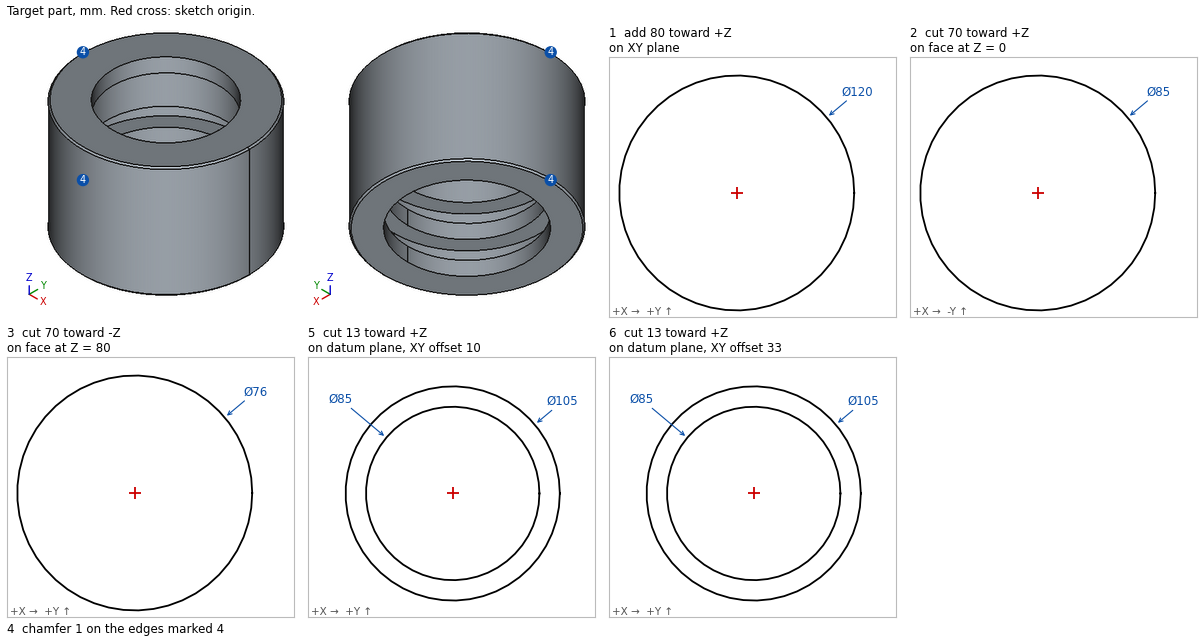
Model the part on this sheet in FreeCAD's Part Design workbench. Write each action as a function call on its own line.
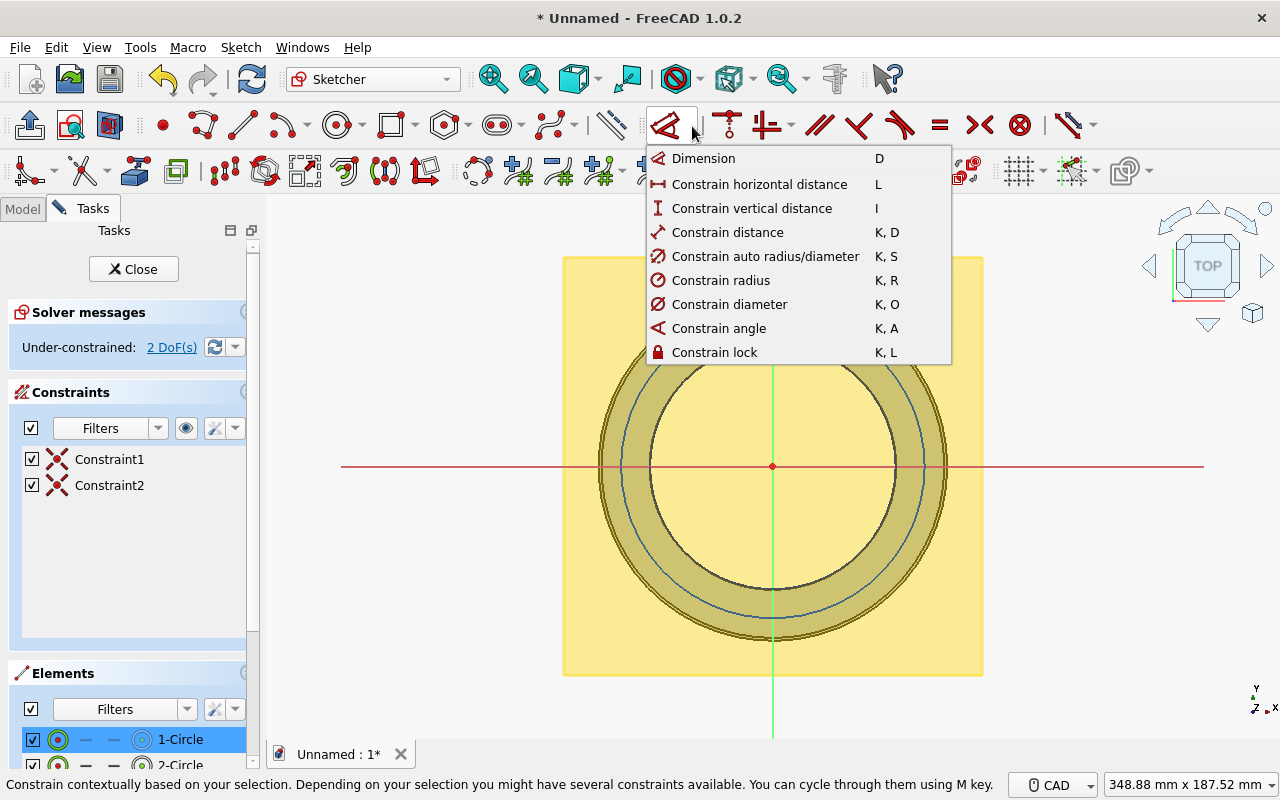
click(799, 304)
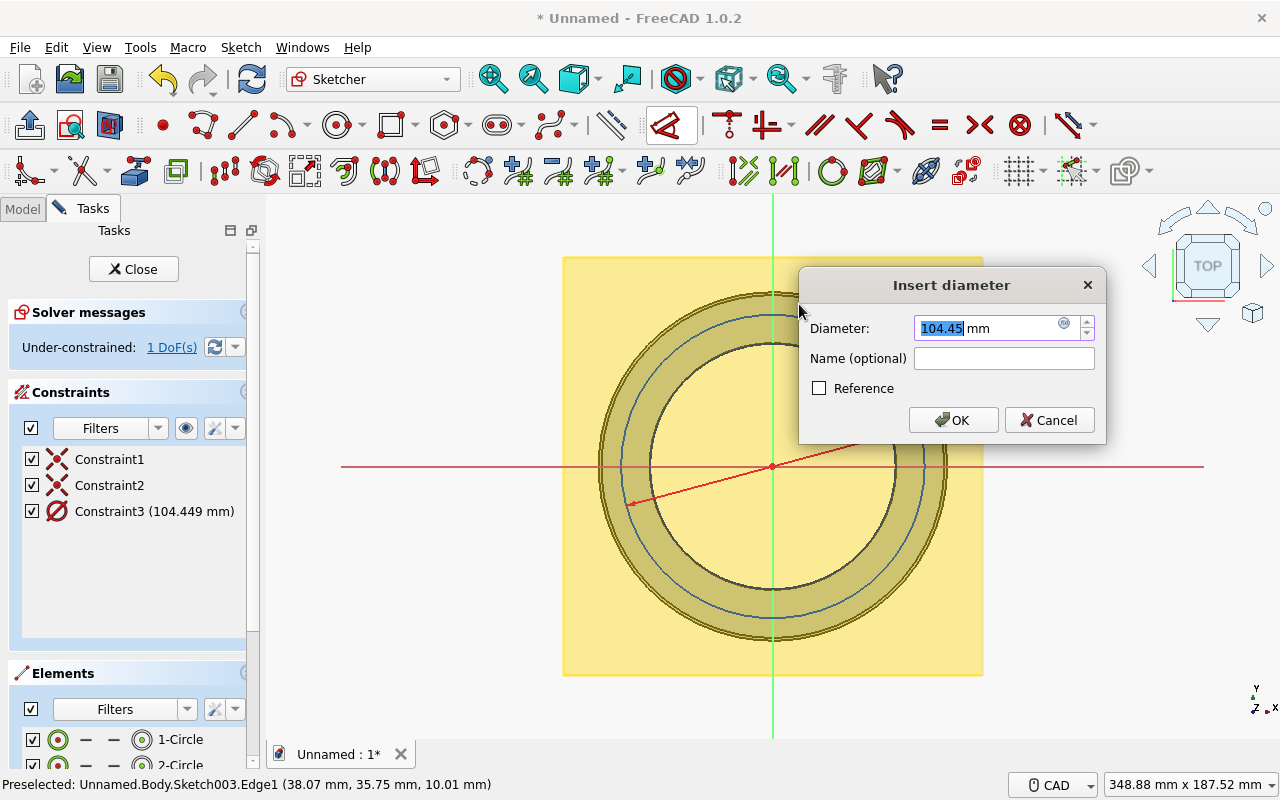
text(105)
key(Return)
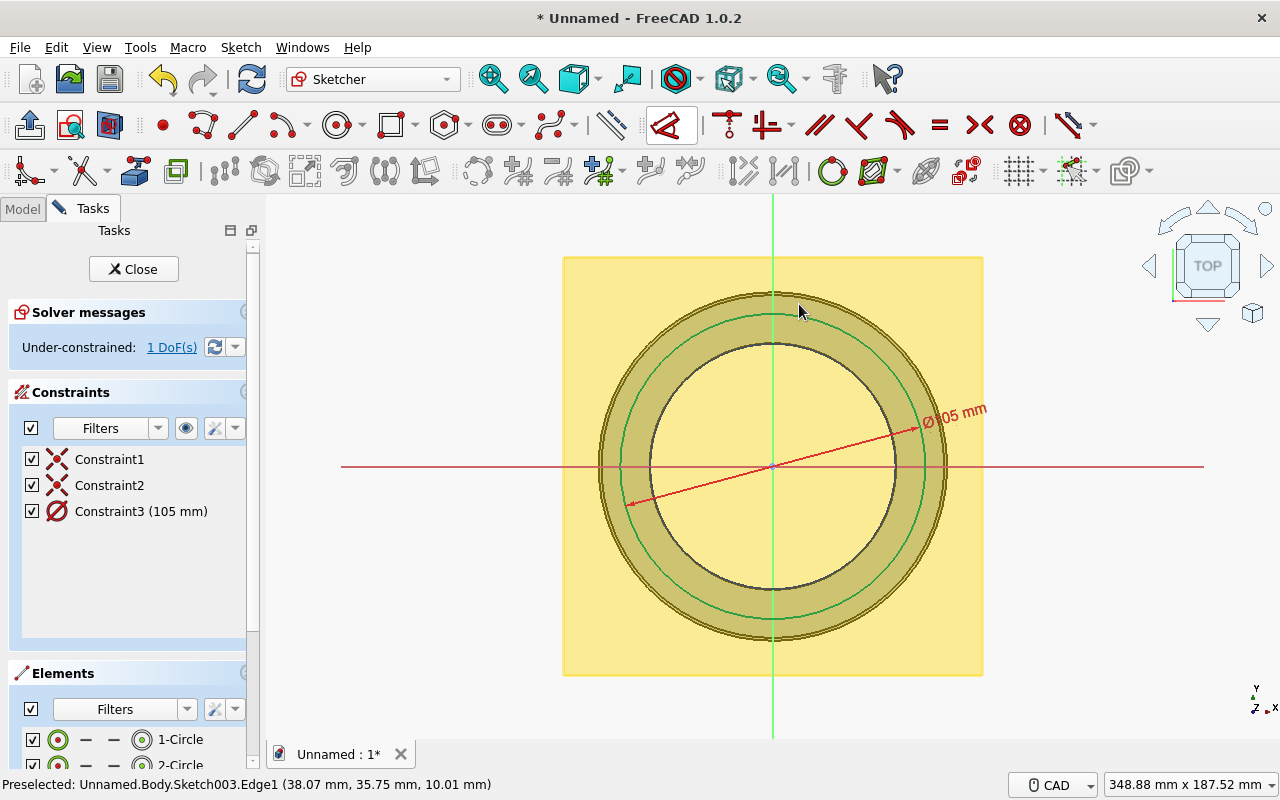
click(859, 379)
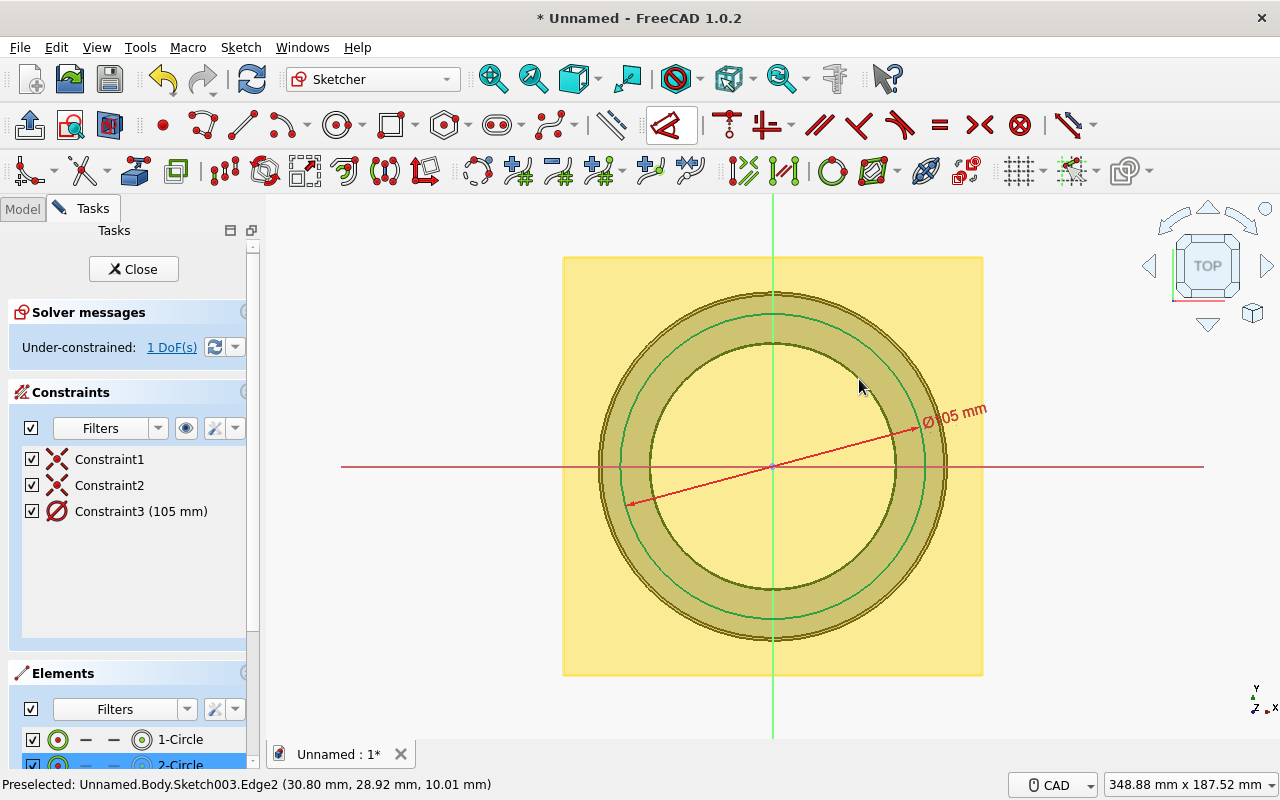
key(k)
key(o)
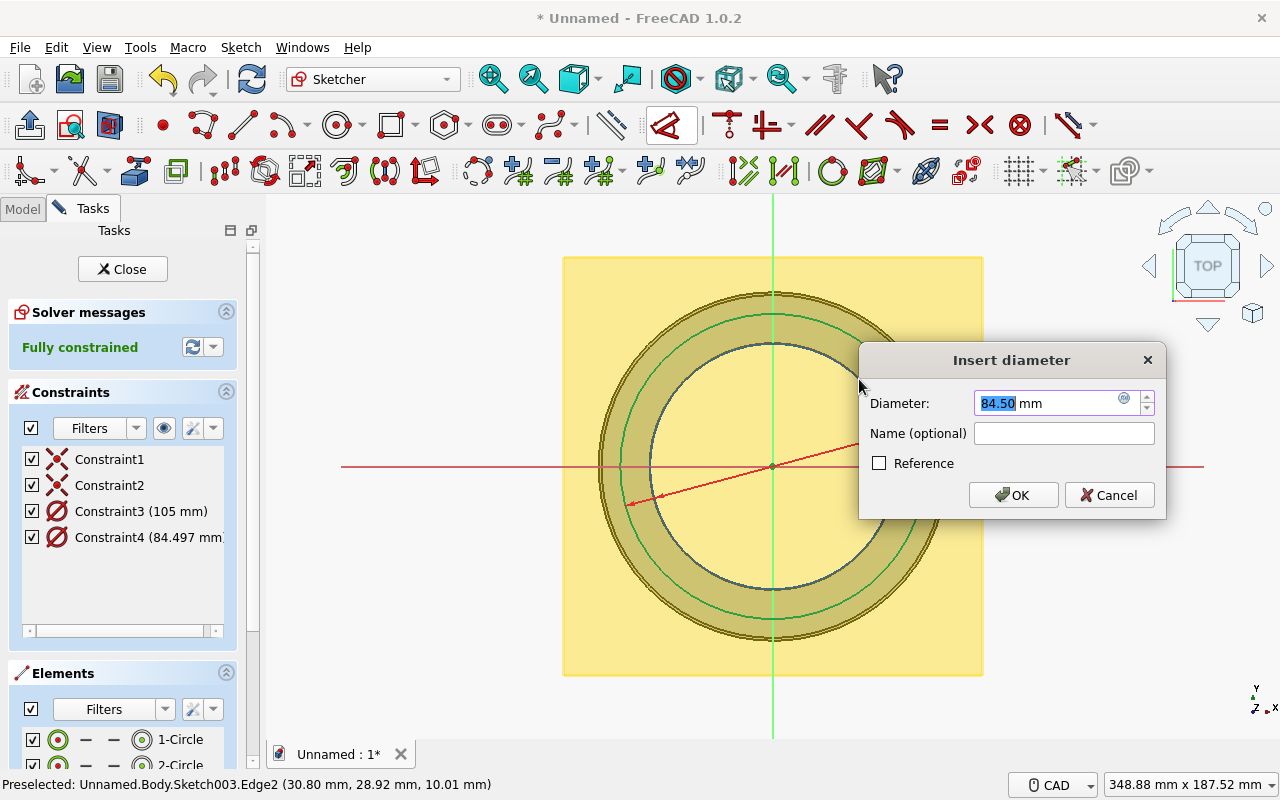
text(85)
key(Return)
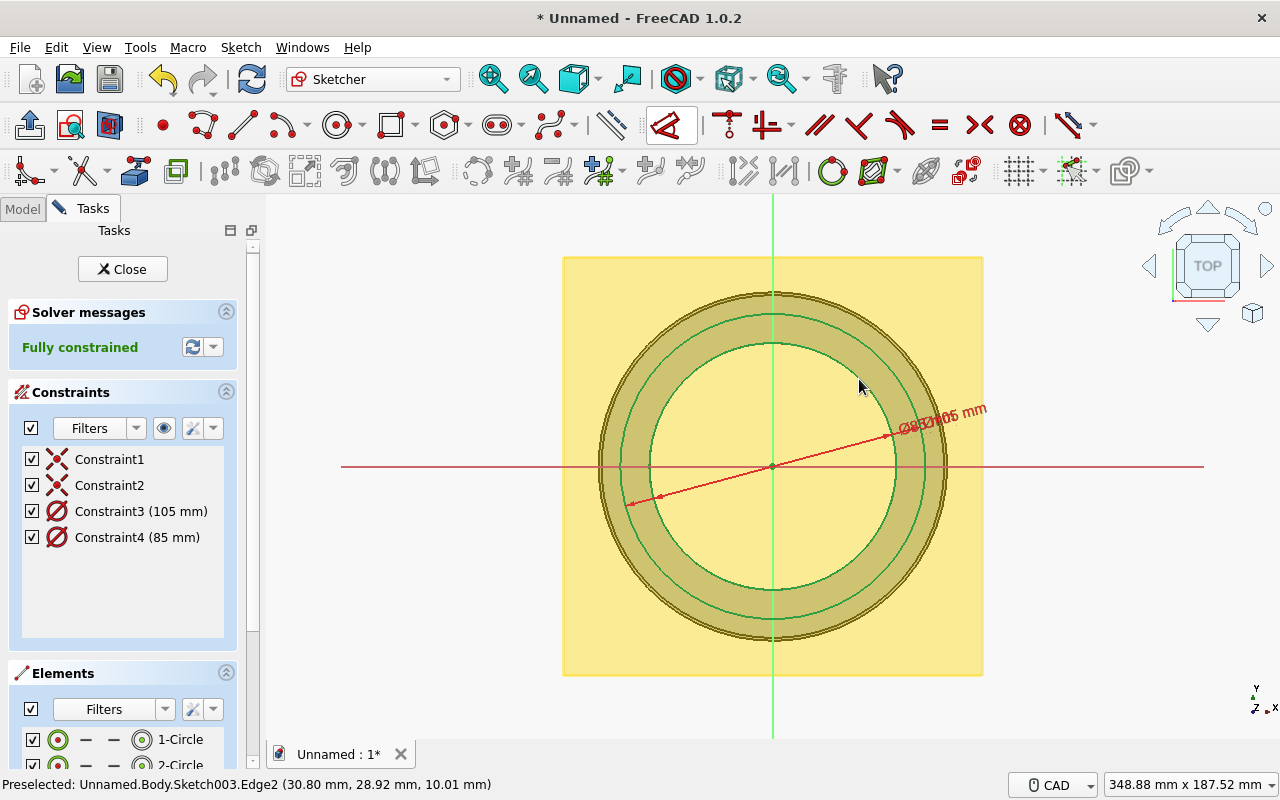
click(123, 269)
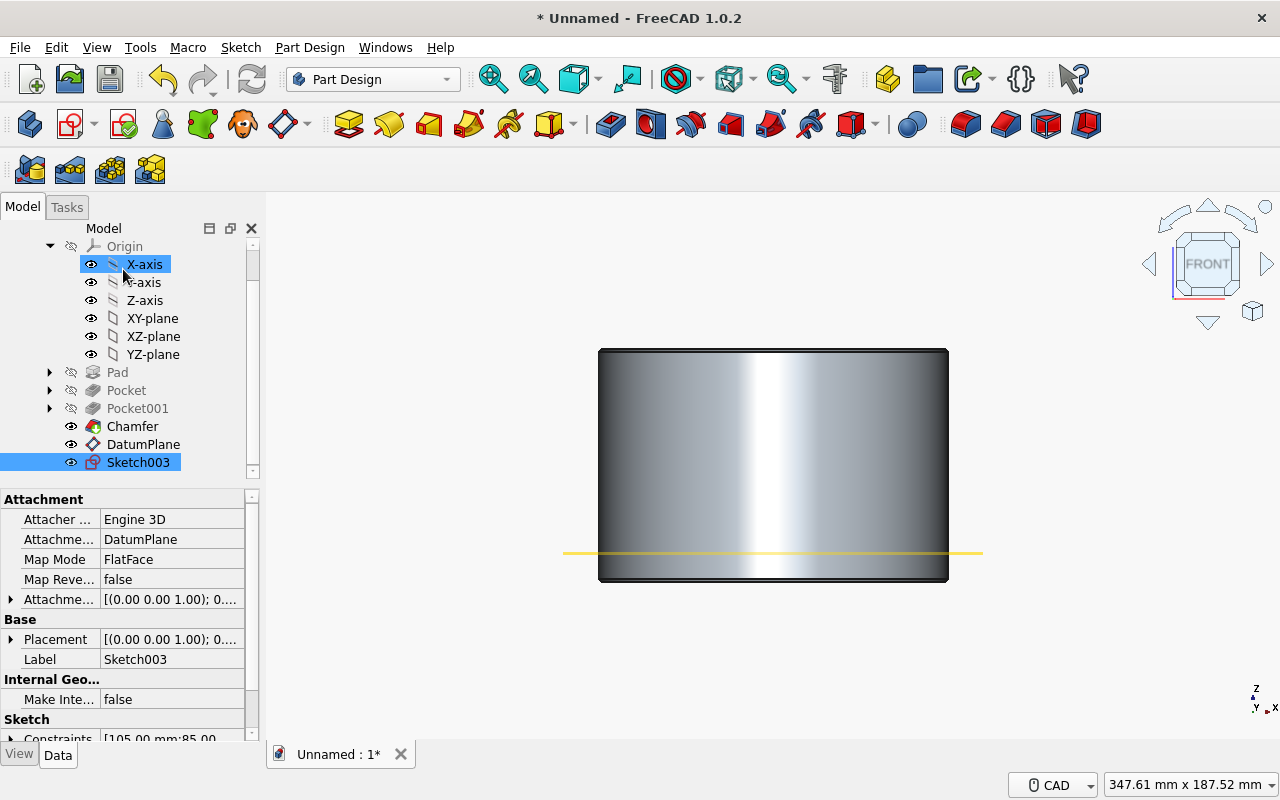
click(612, 124)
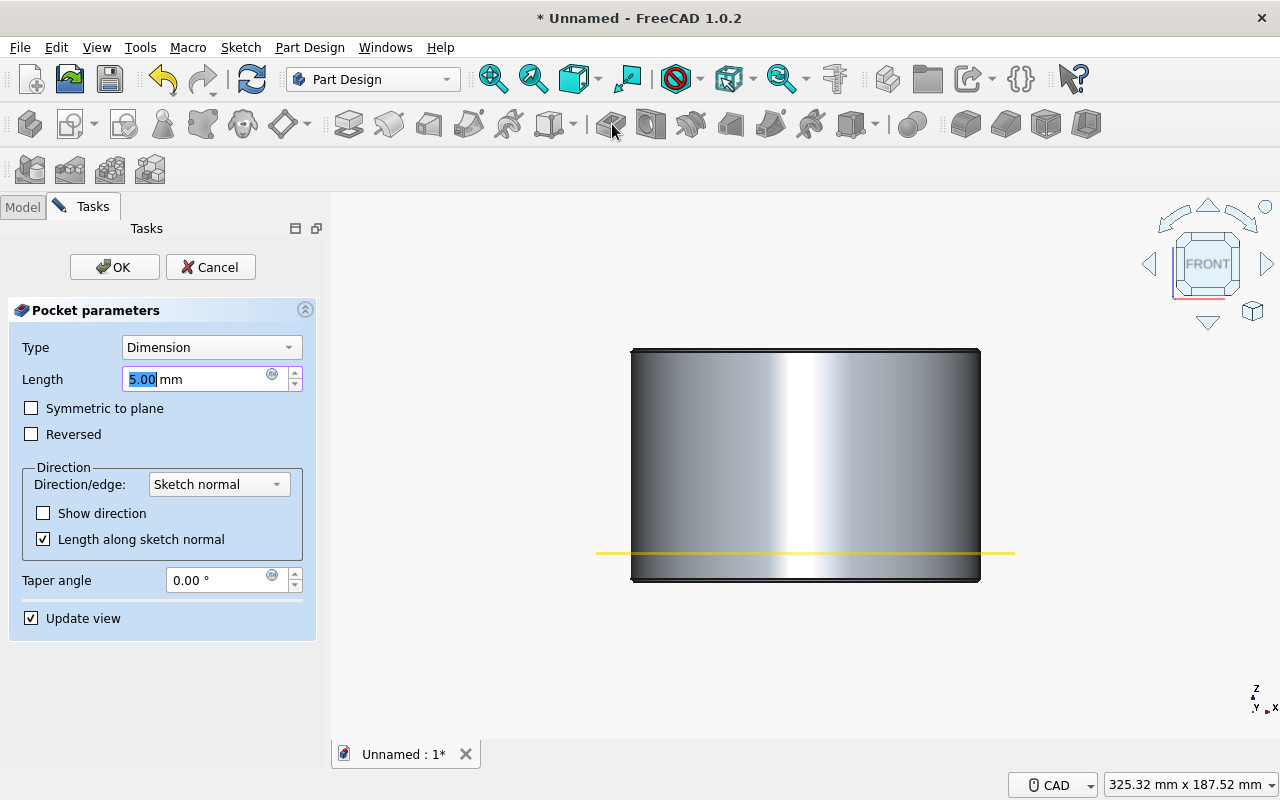
text(13)
key(Tab)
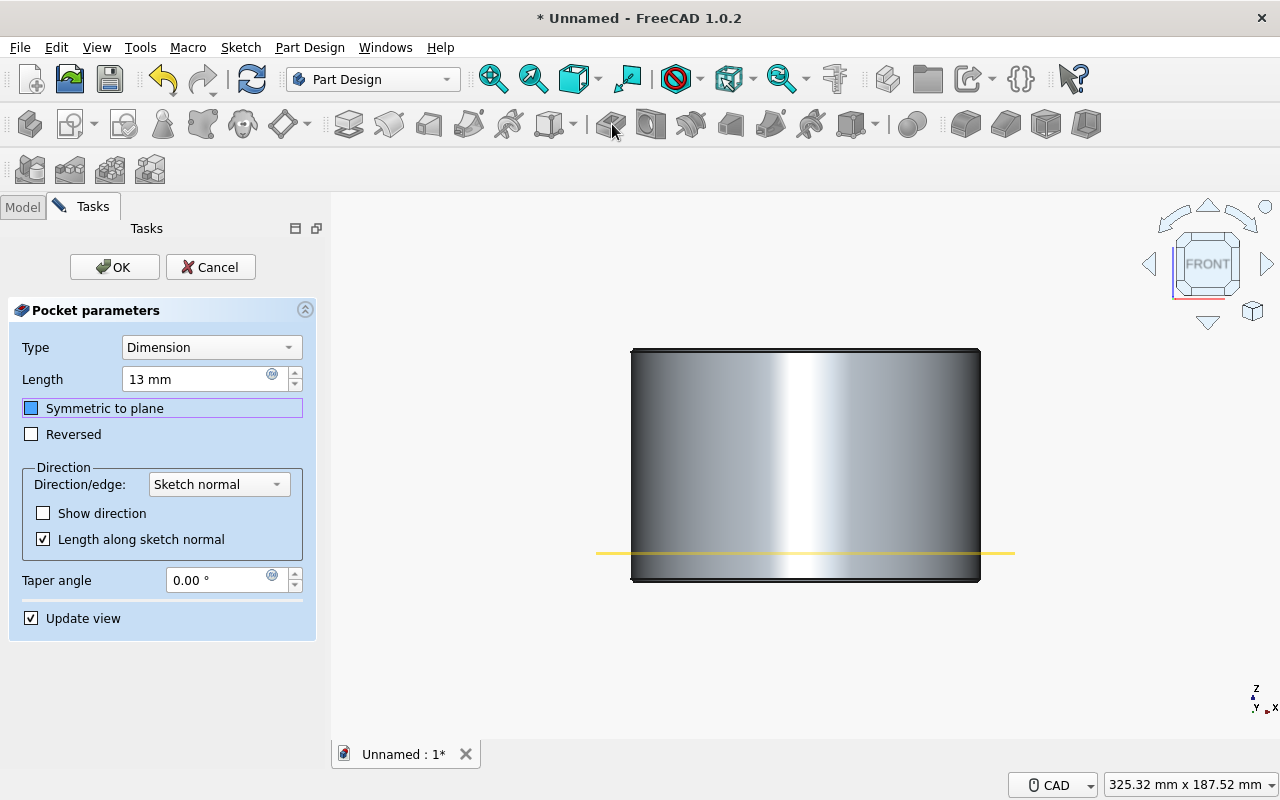
click(30, 434)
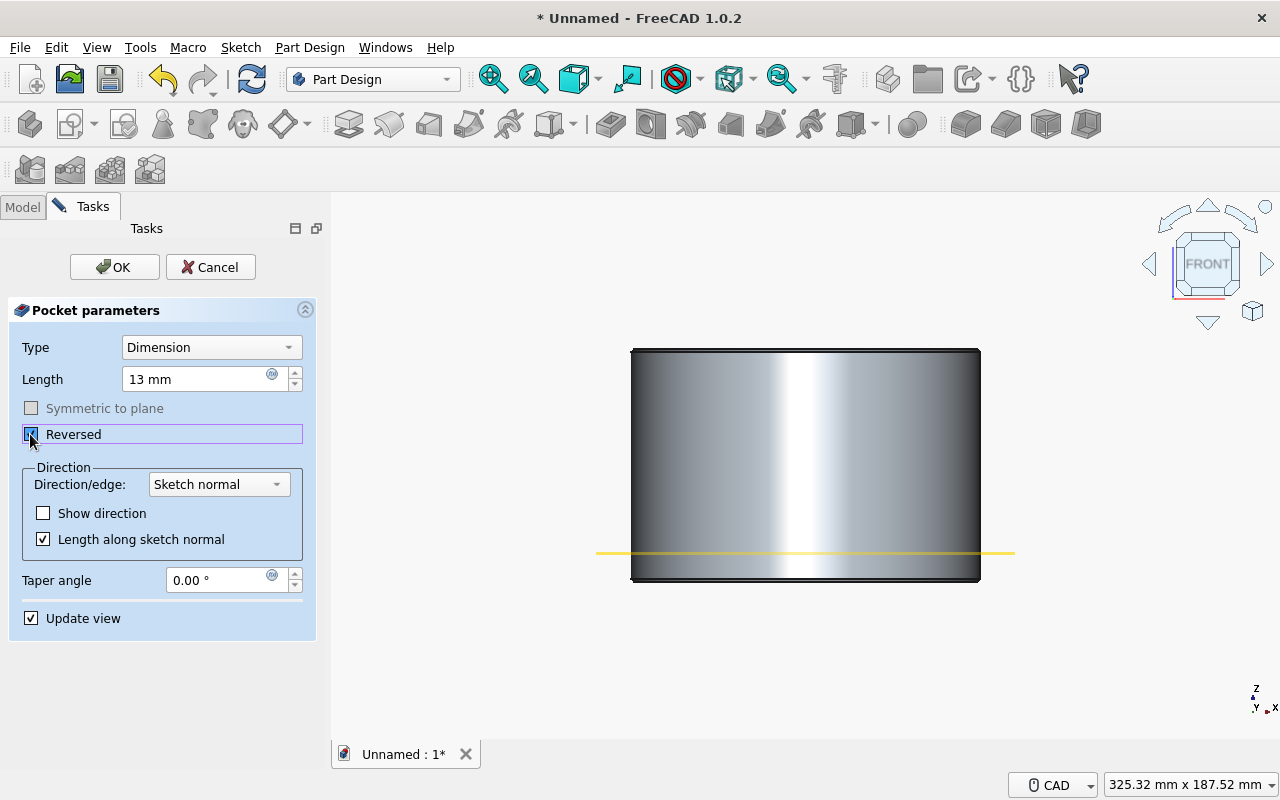
click(115, 267)